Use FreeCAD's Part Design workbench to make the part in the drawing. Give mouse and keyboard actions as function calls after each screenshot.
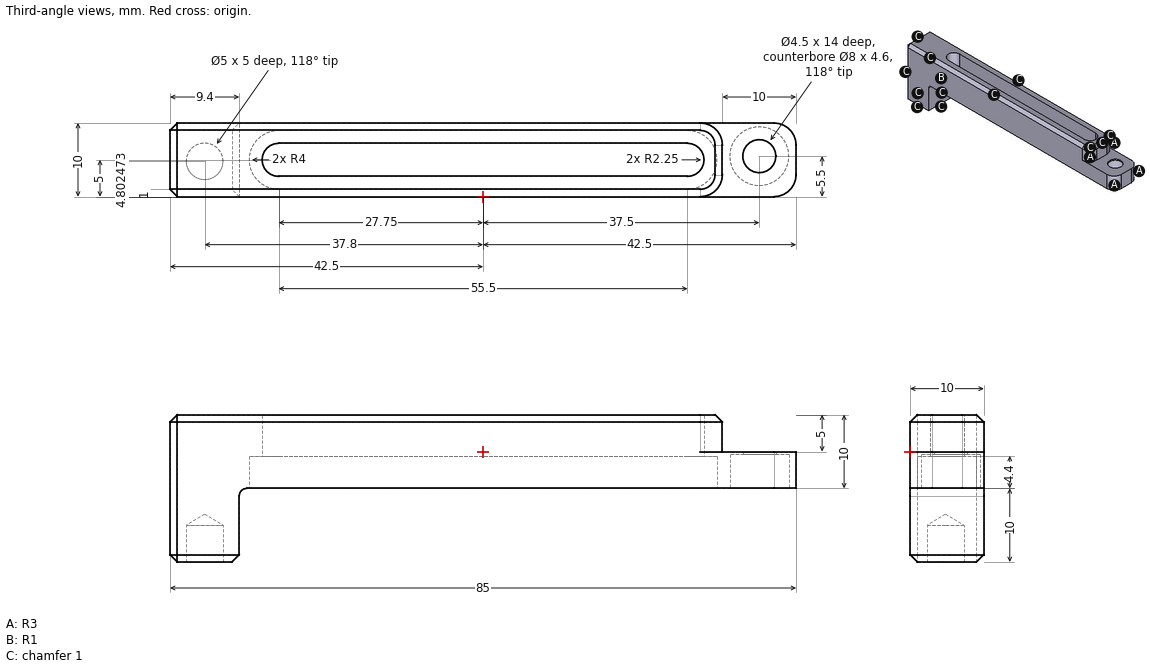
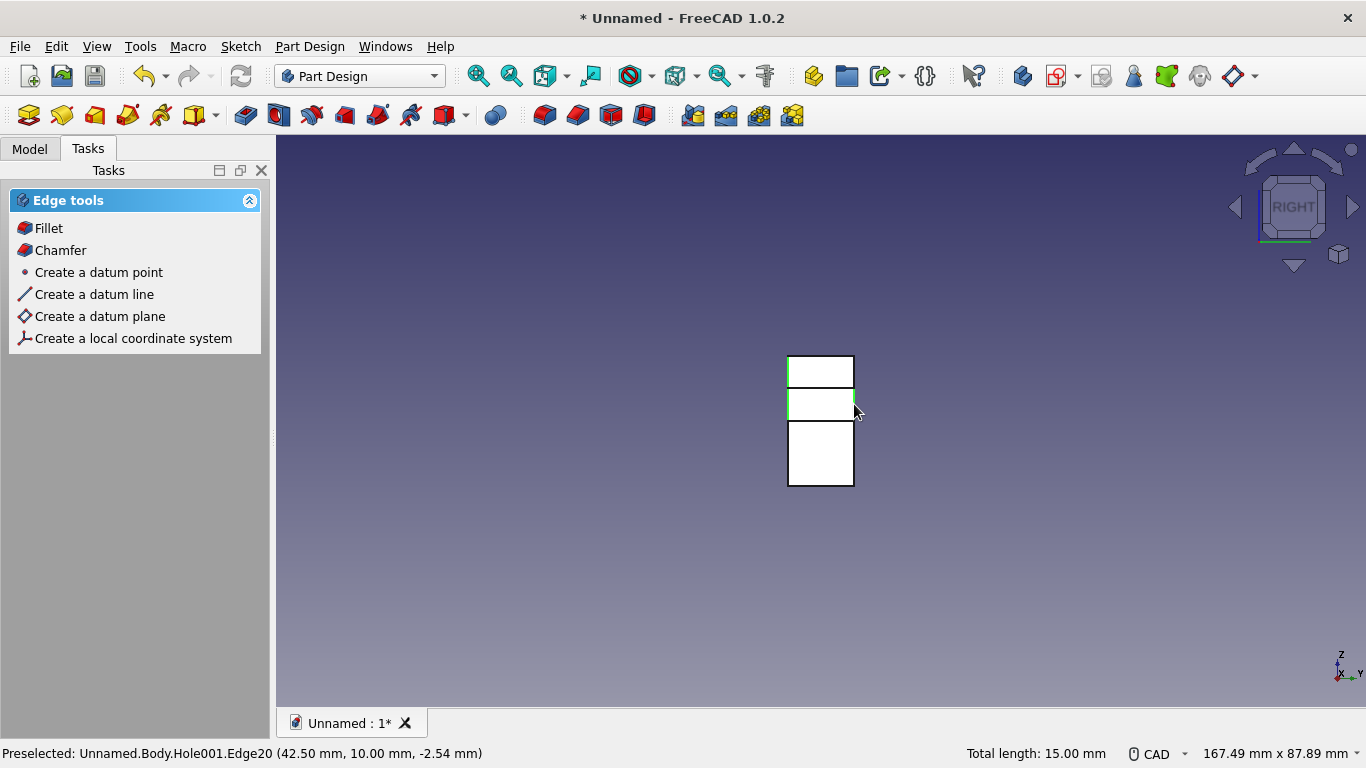
click(854, 371, ctrl)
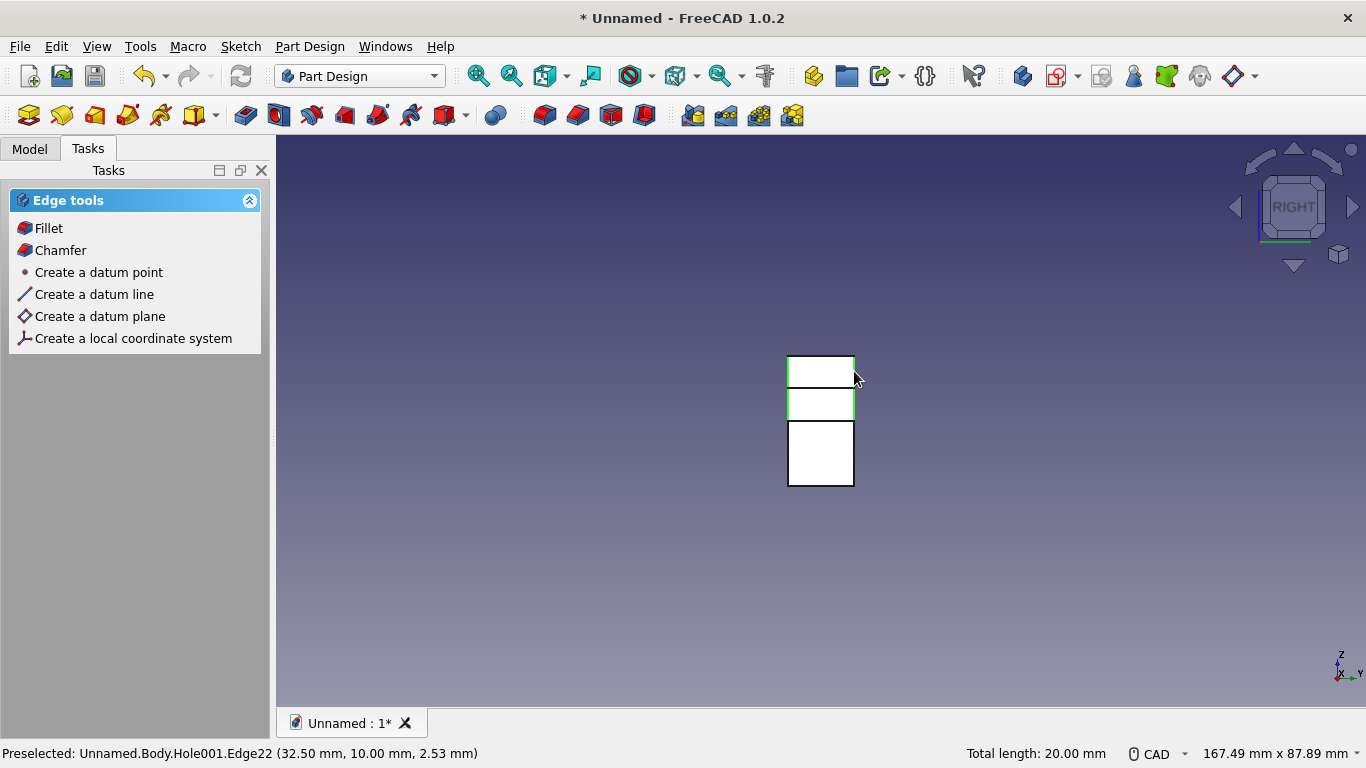
click(545, 116)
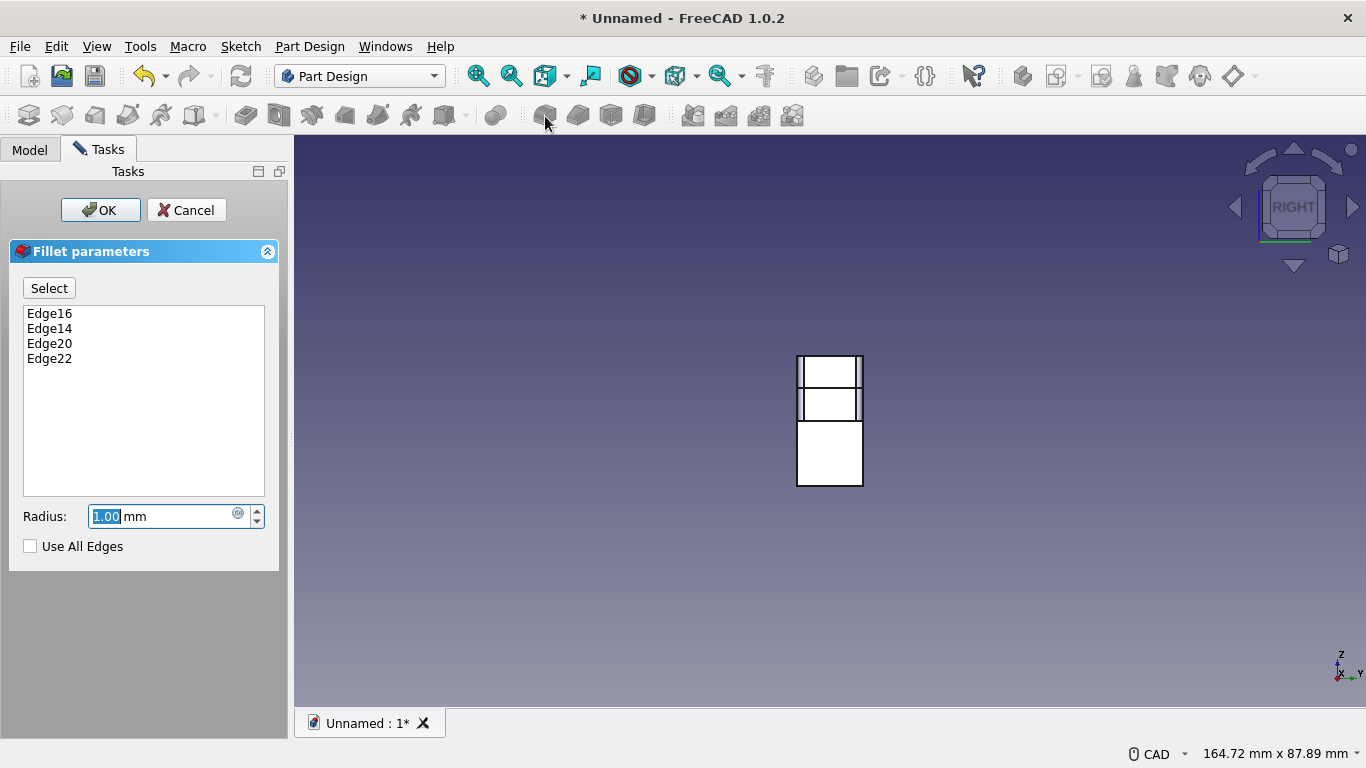
text(3)
key(Tab)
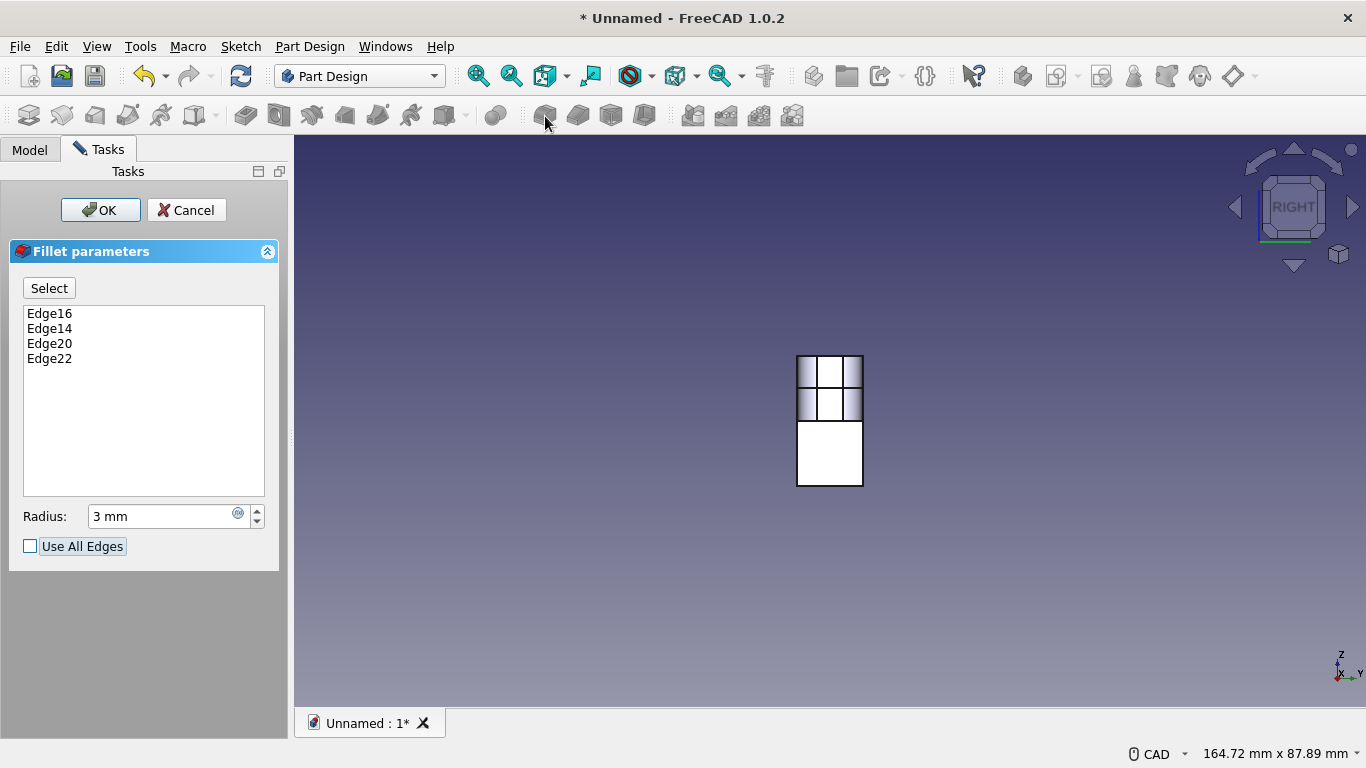
click(101, 210)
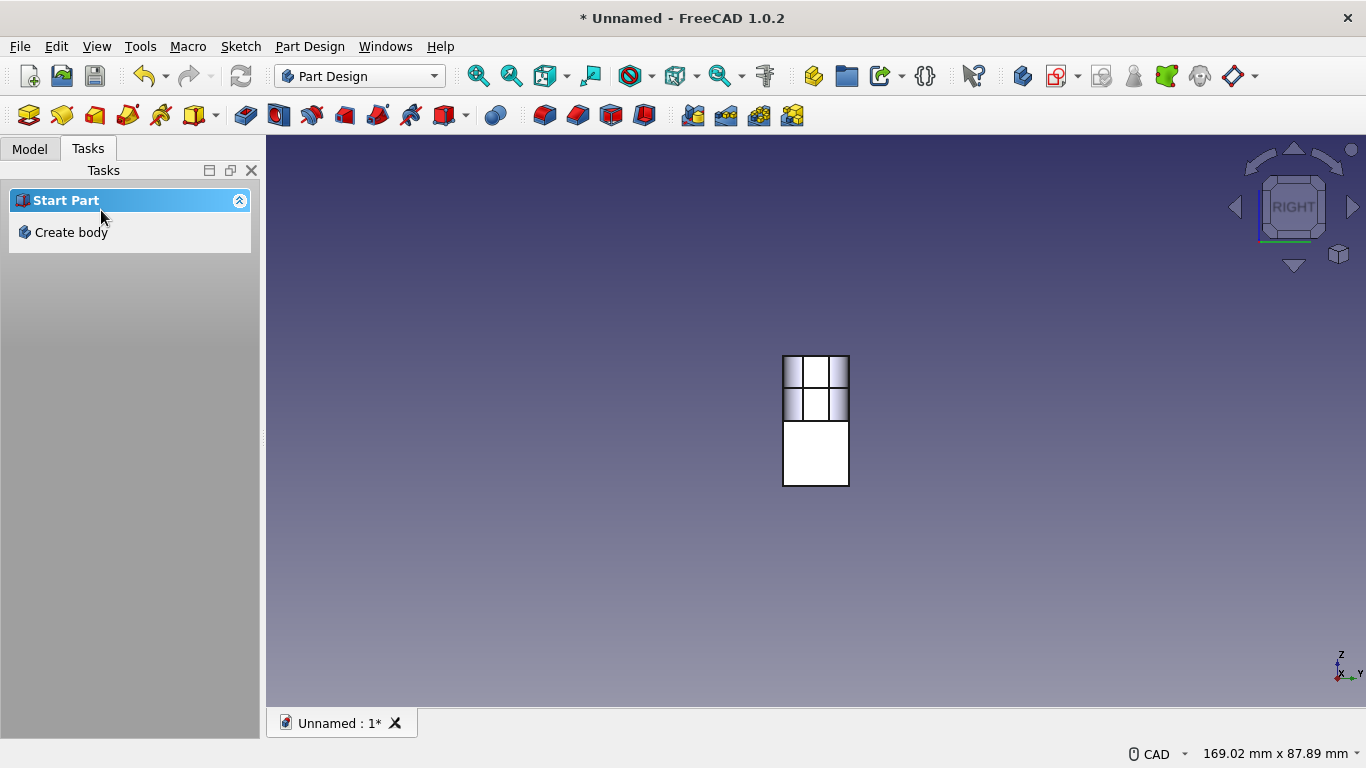
key(v)
key(f)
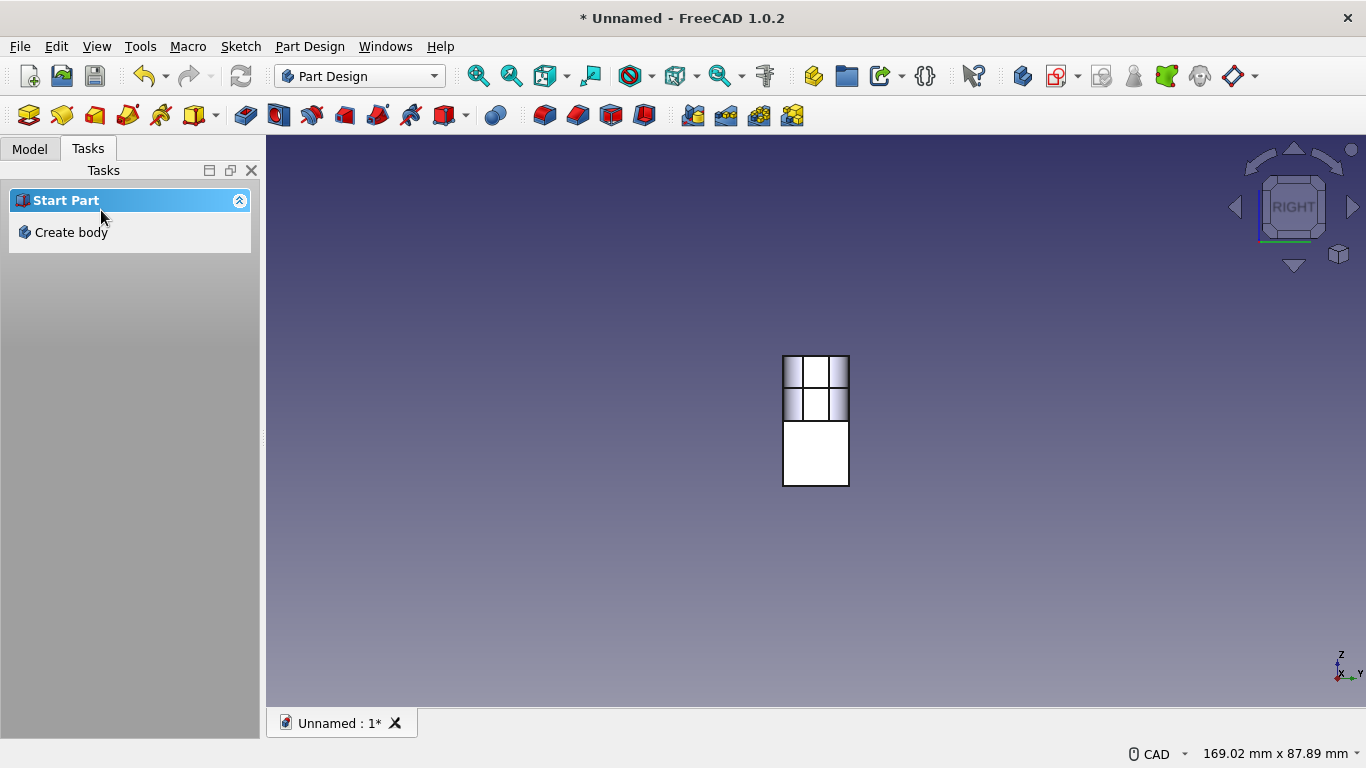
key(0)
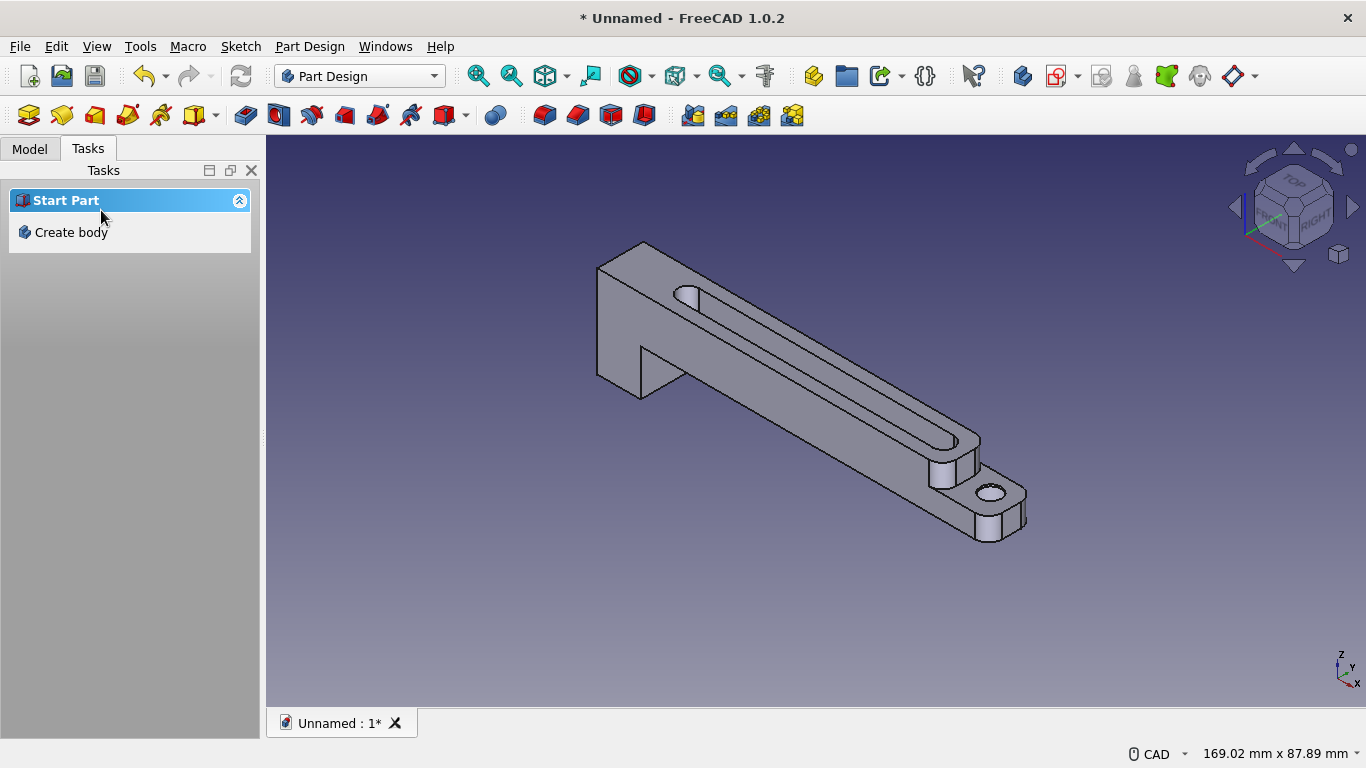
key(2)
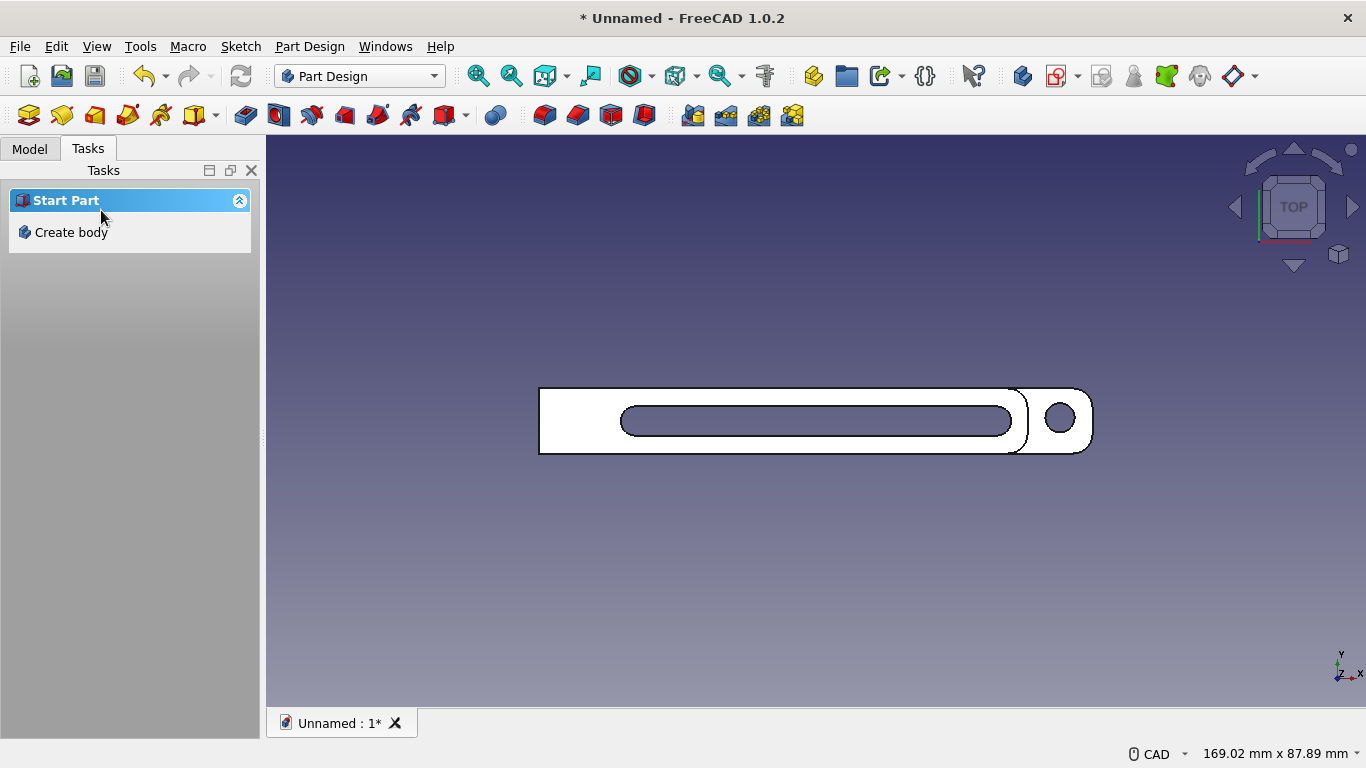
key(1)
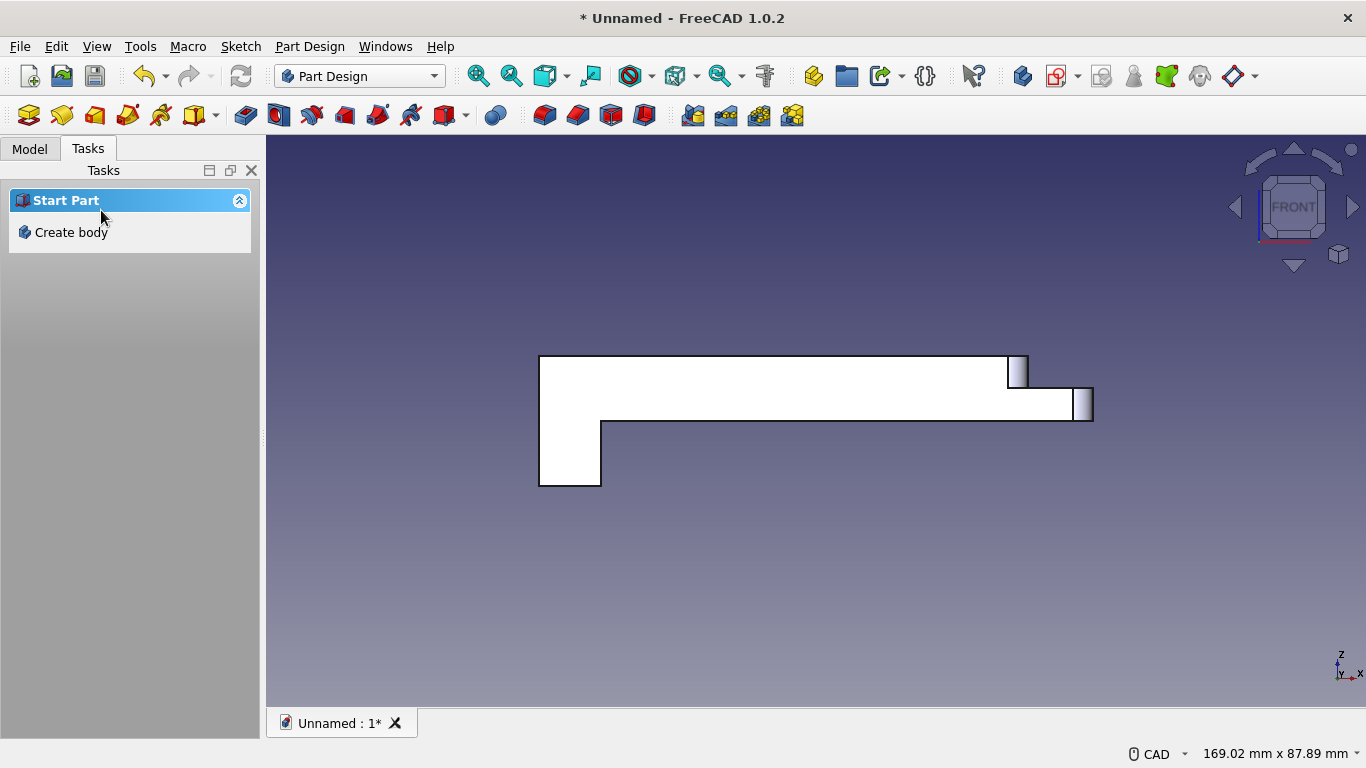
key(3)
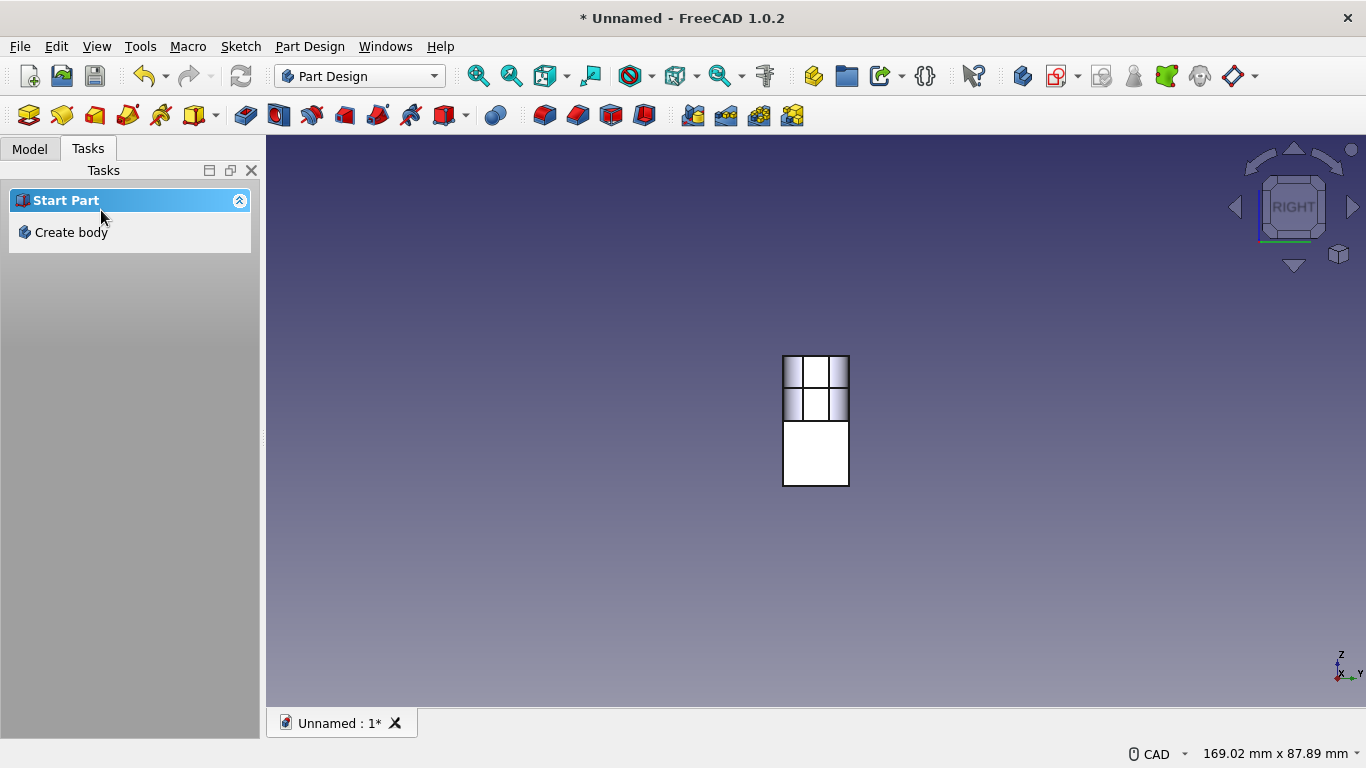
key(v)
key(f)